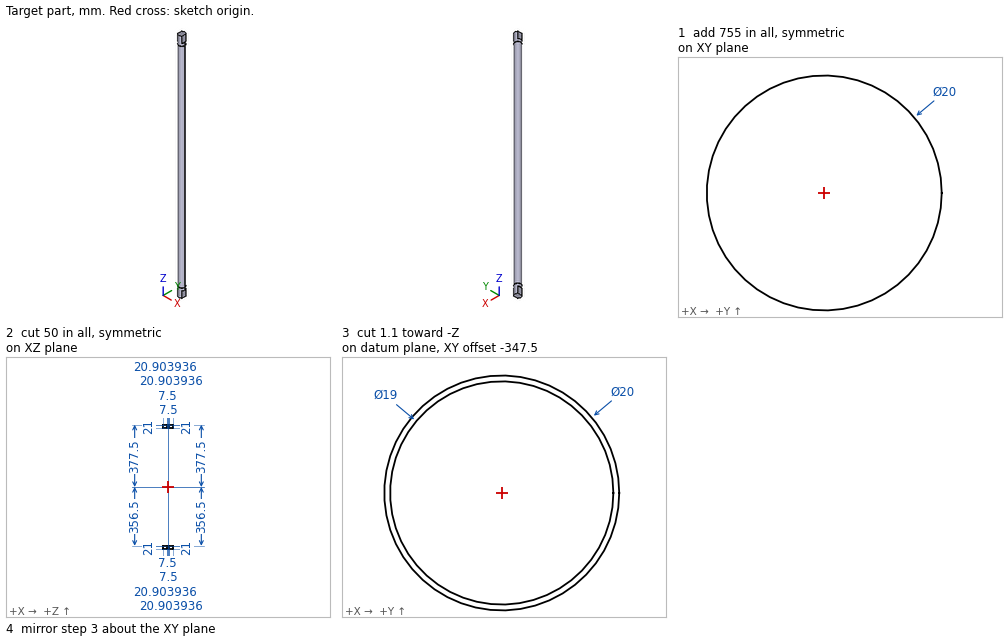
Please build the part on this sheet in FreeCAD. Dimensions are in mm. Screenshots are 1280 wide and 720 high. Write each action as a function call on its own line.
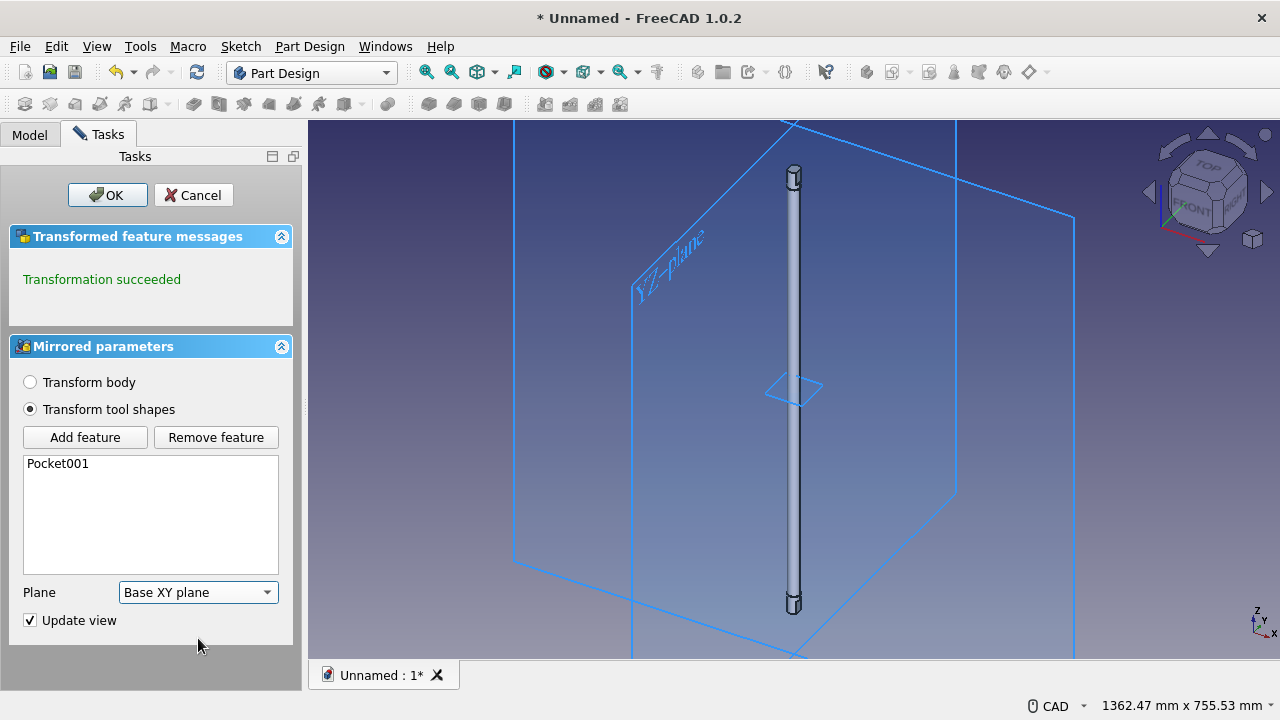
click(108, 195)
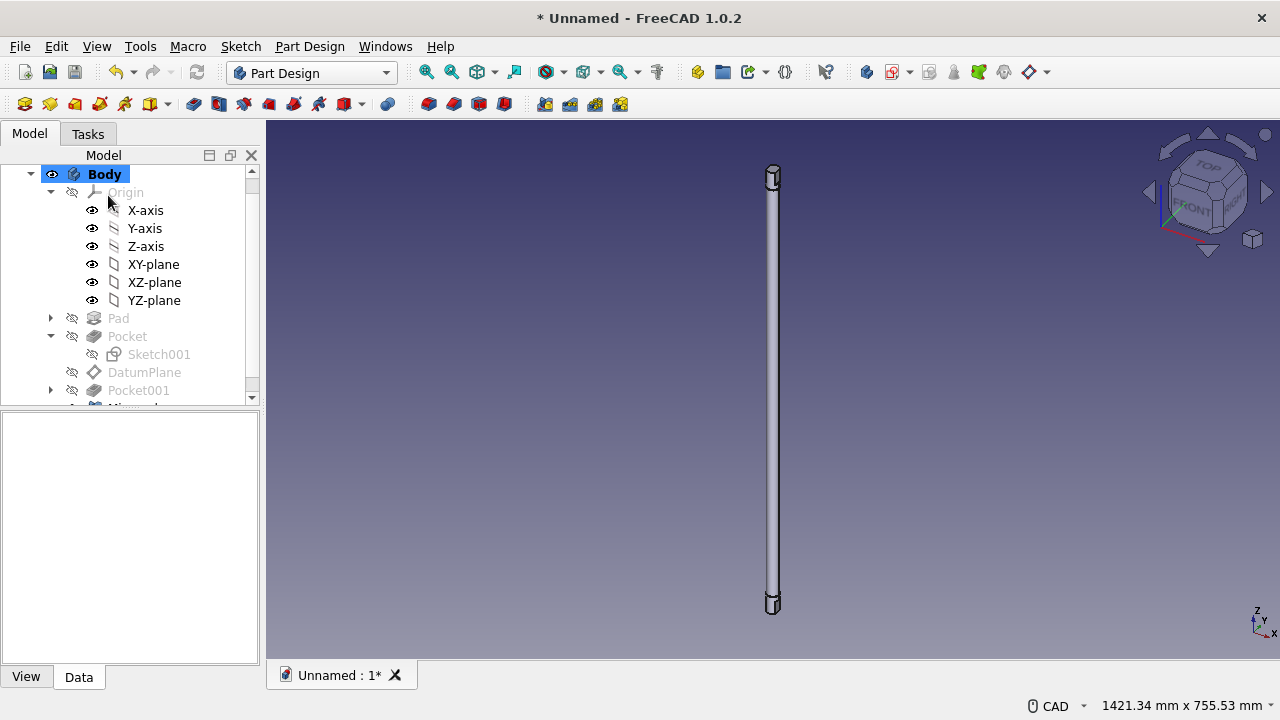
key(0)